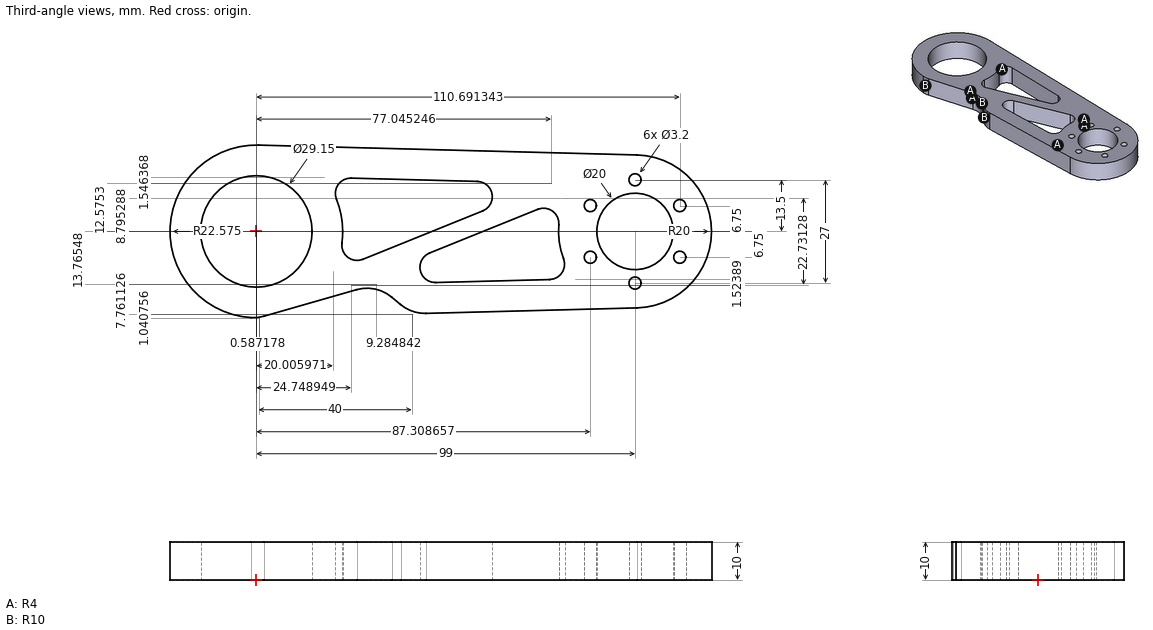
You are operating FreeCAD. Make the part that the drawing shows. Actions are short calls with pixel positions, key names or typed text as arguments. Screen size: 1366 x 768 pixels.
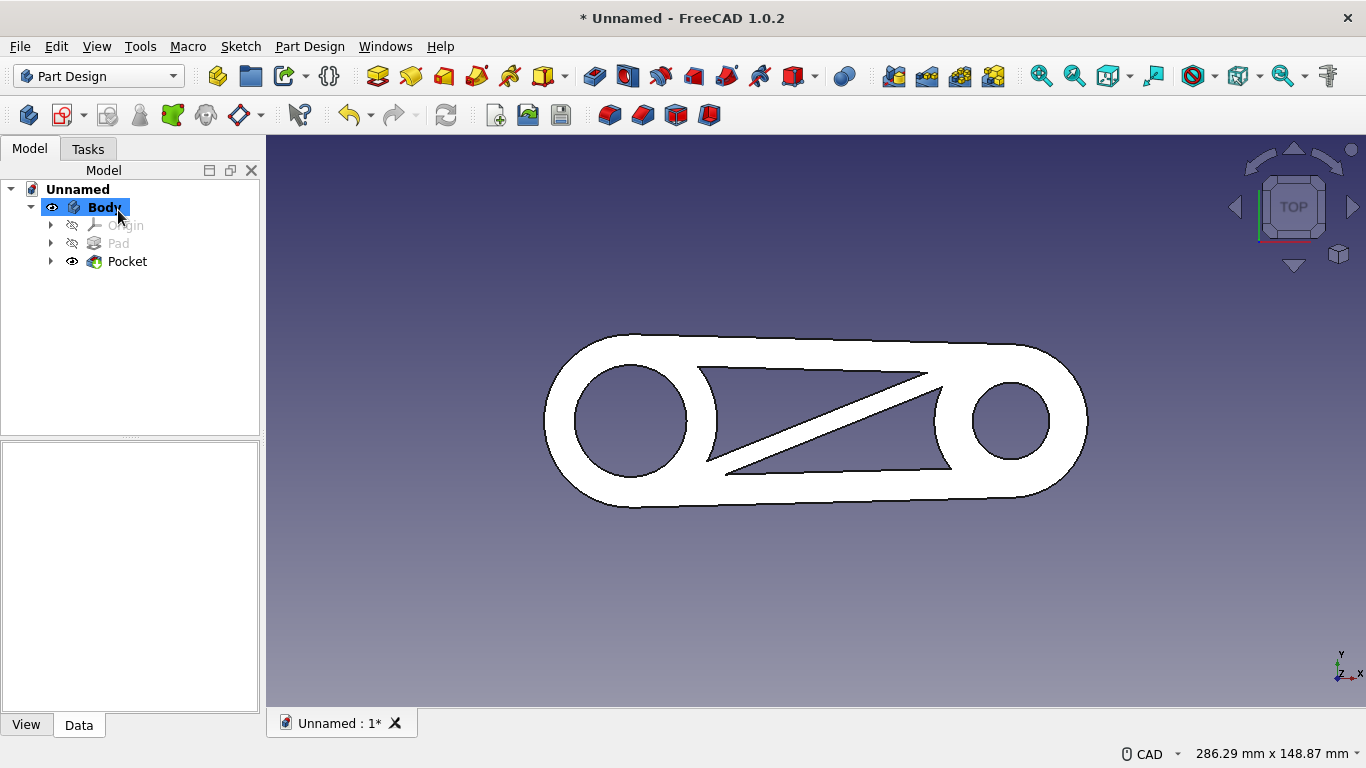
key(1)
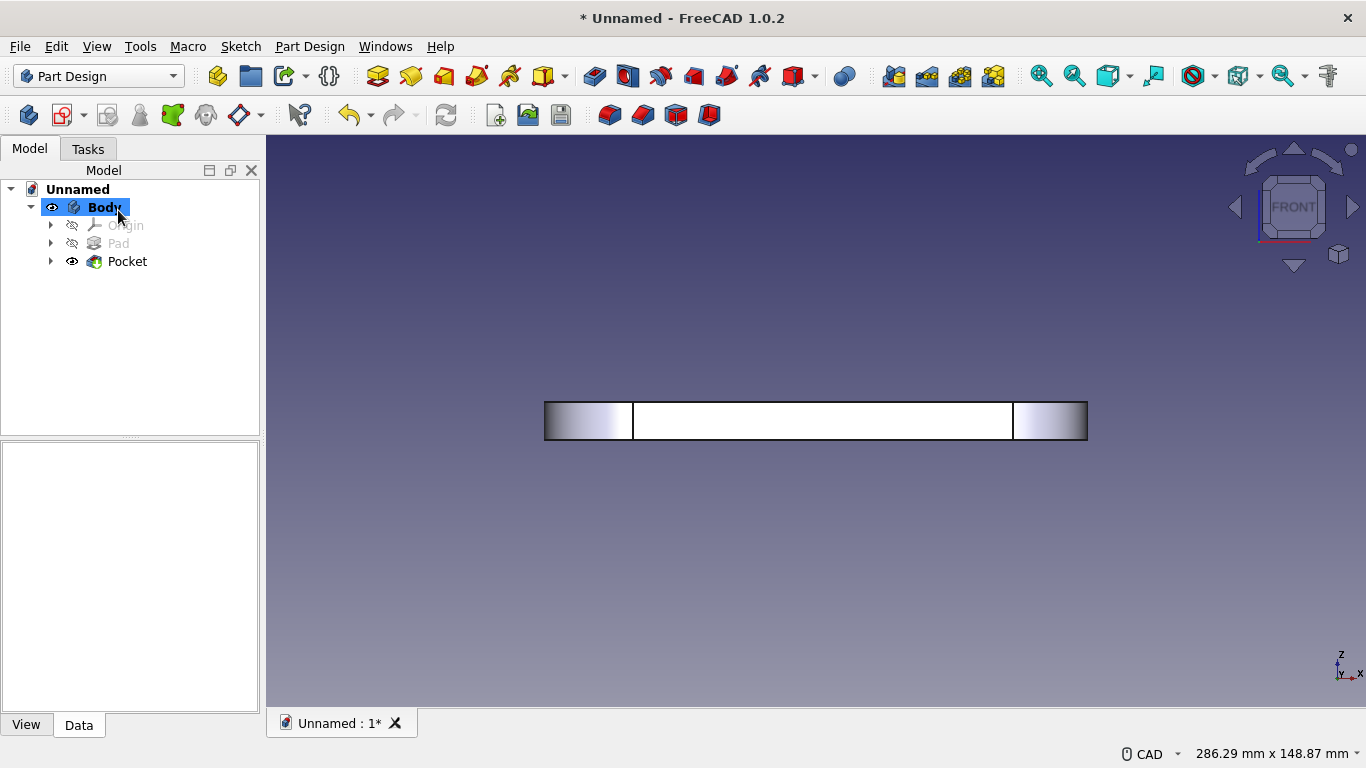
key(3)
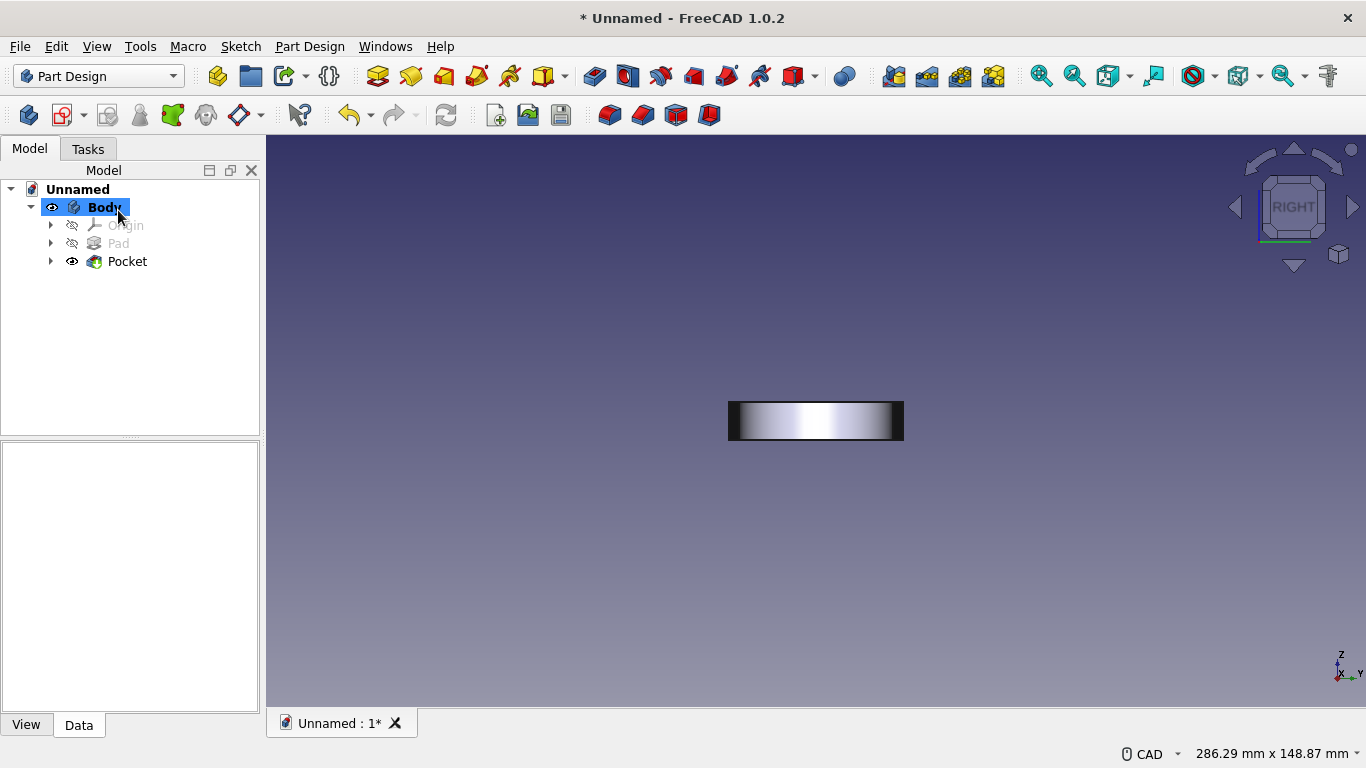
click(1042, 76)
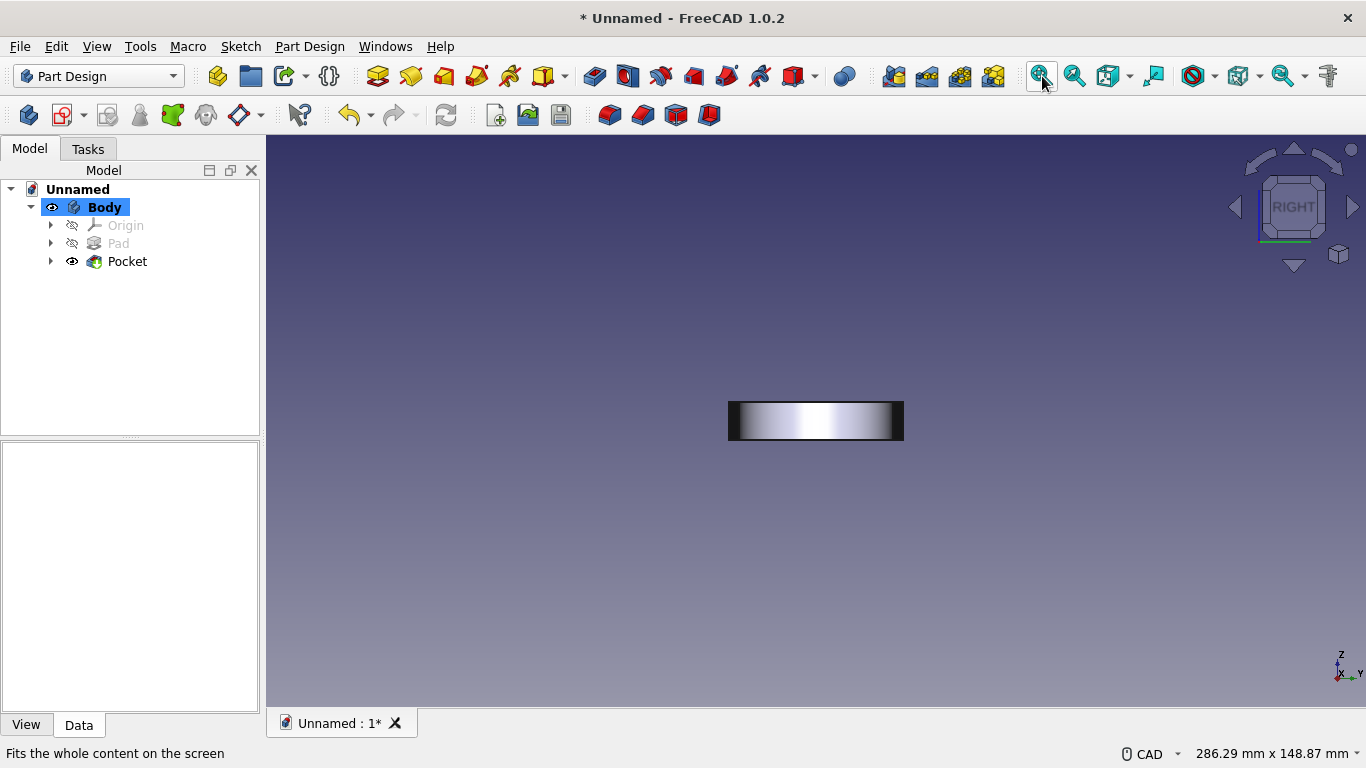
key(5)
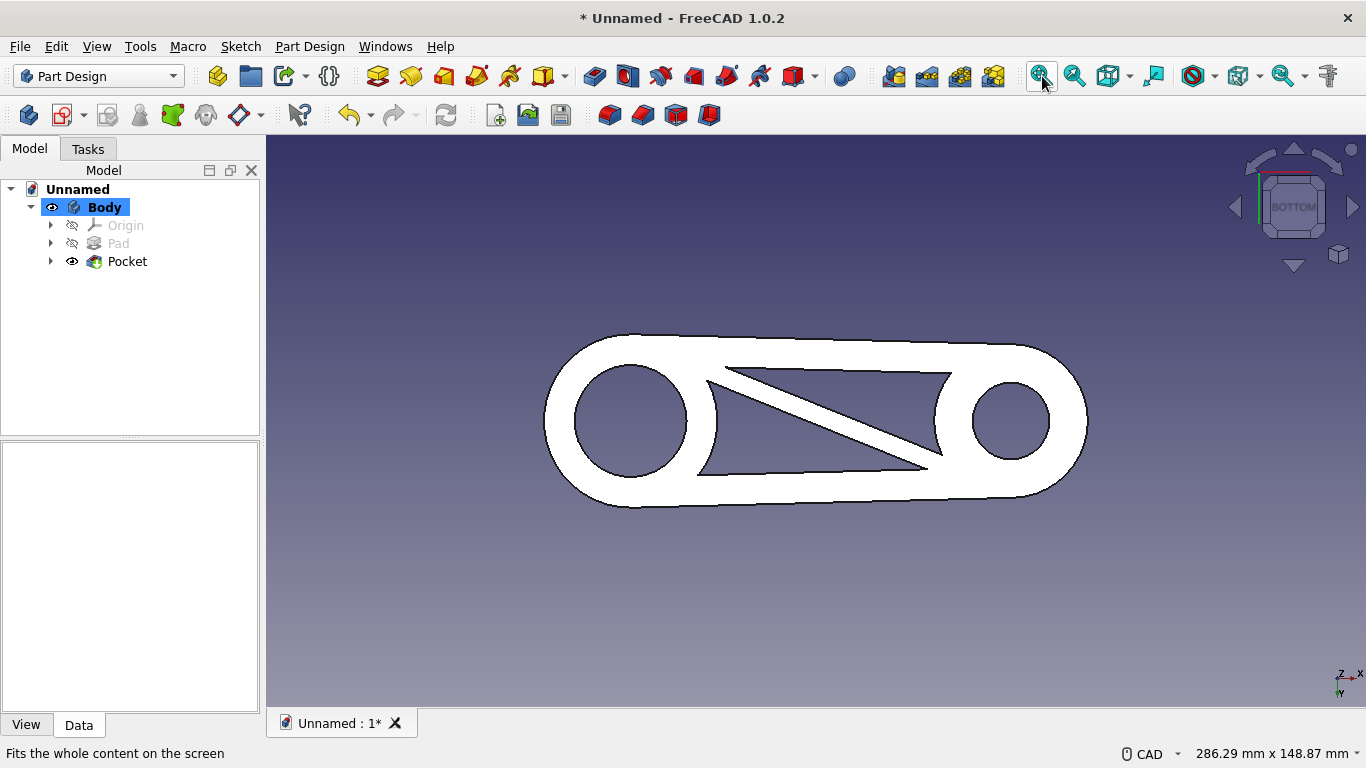
key(4)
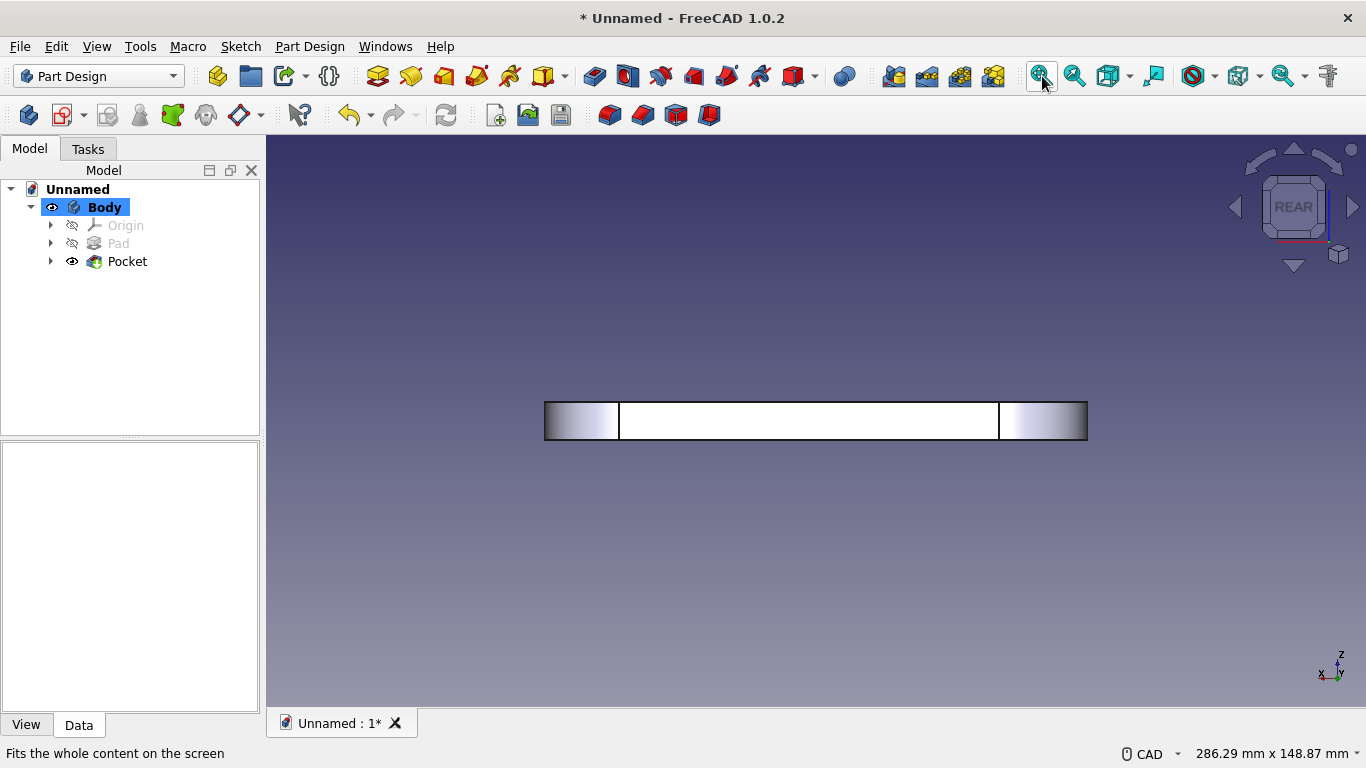
key(6)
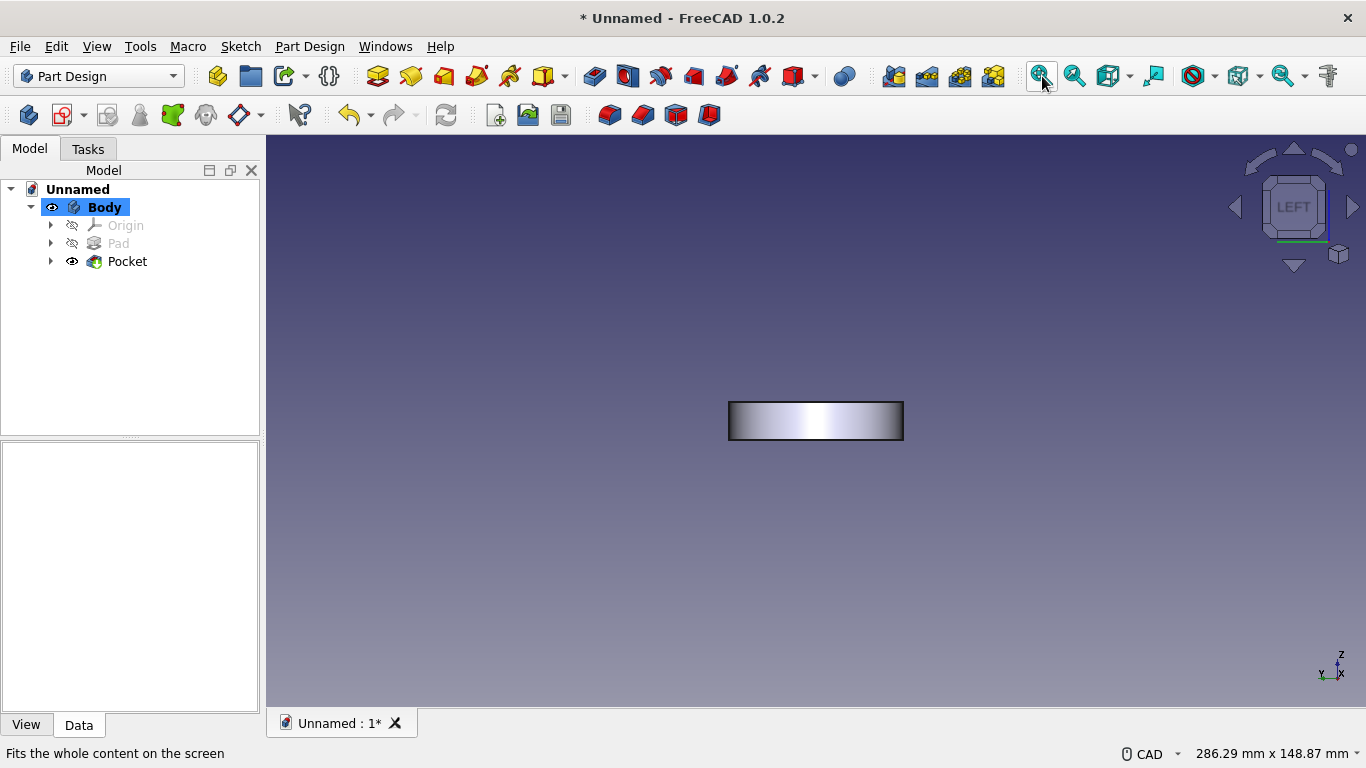
click(1042, 76)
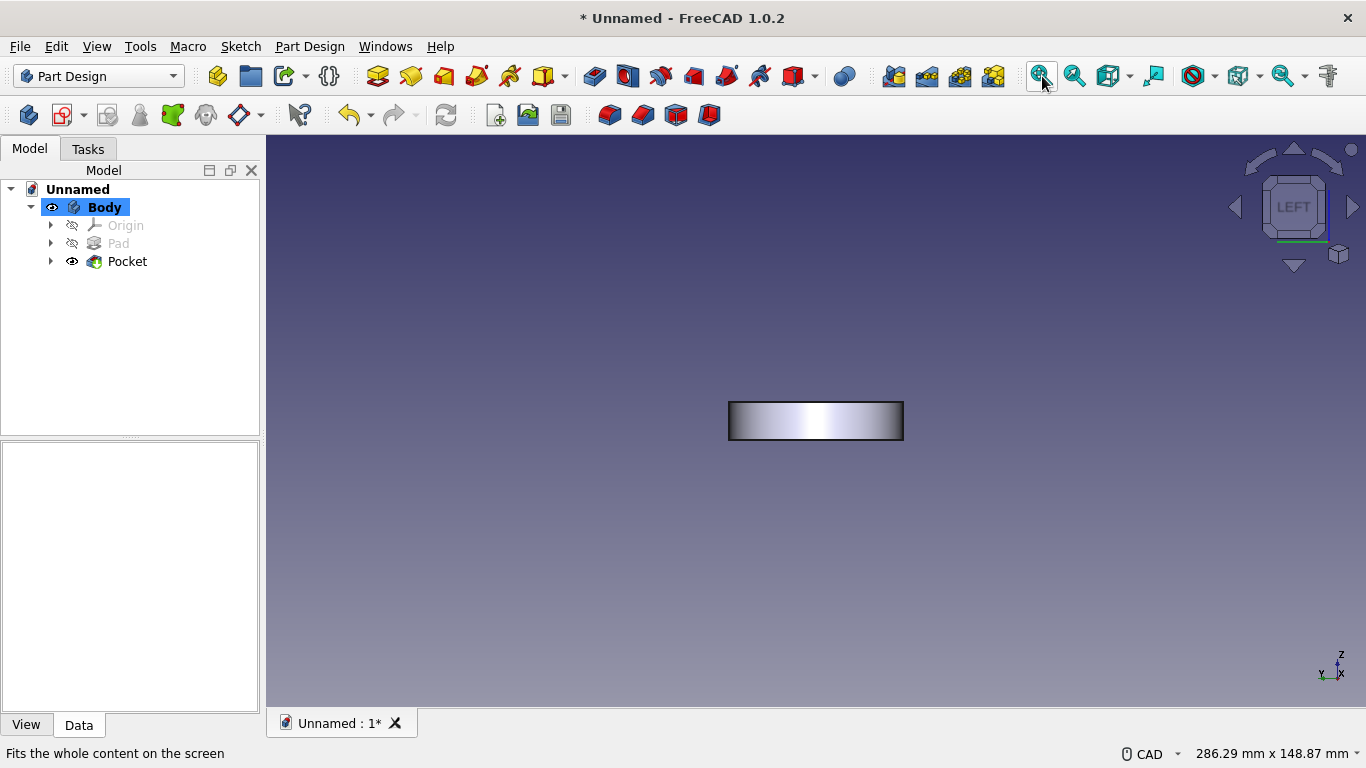
key(v)
key(3)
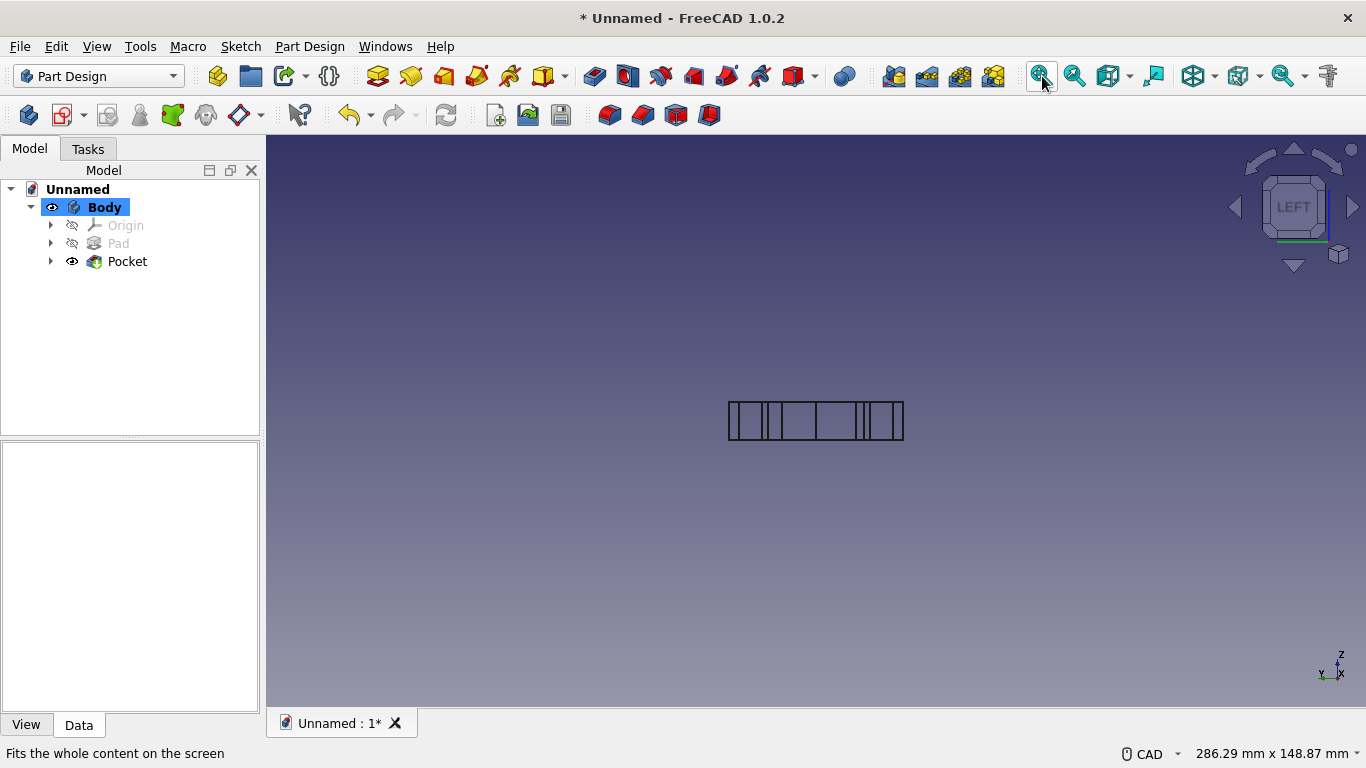
key(0)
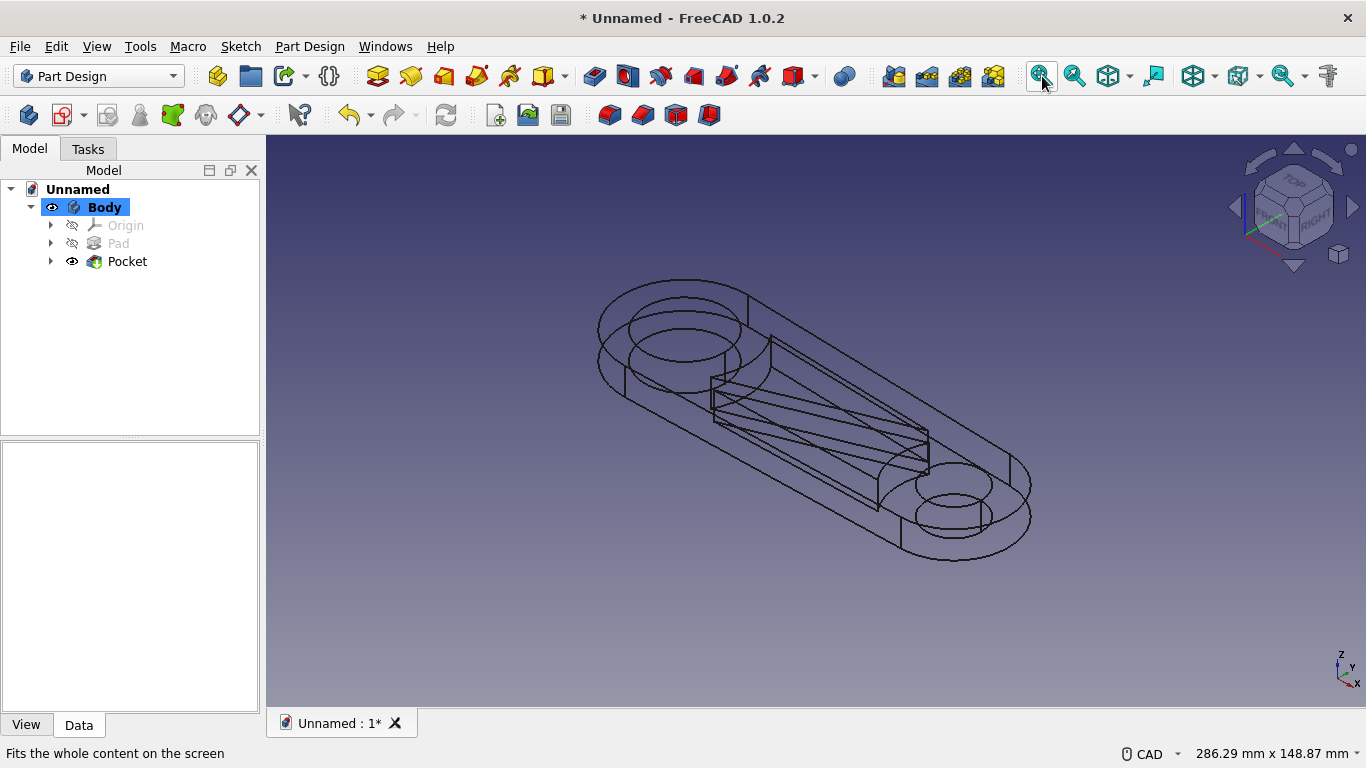
click(929, 458)